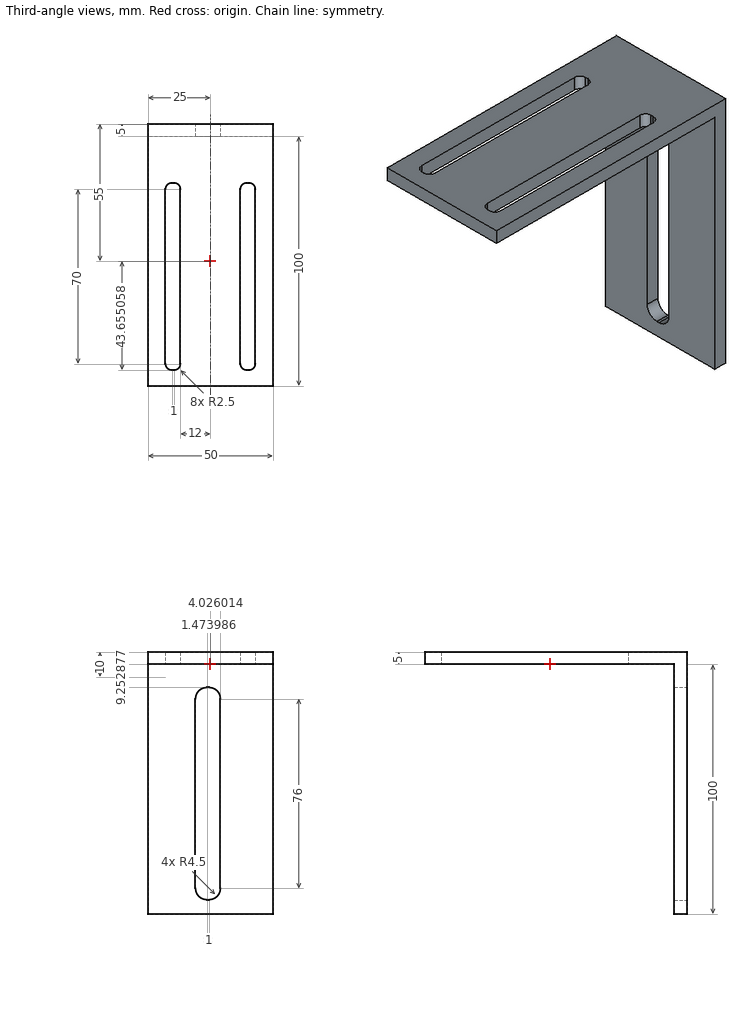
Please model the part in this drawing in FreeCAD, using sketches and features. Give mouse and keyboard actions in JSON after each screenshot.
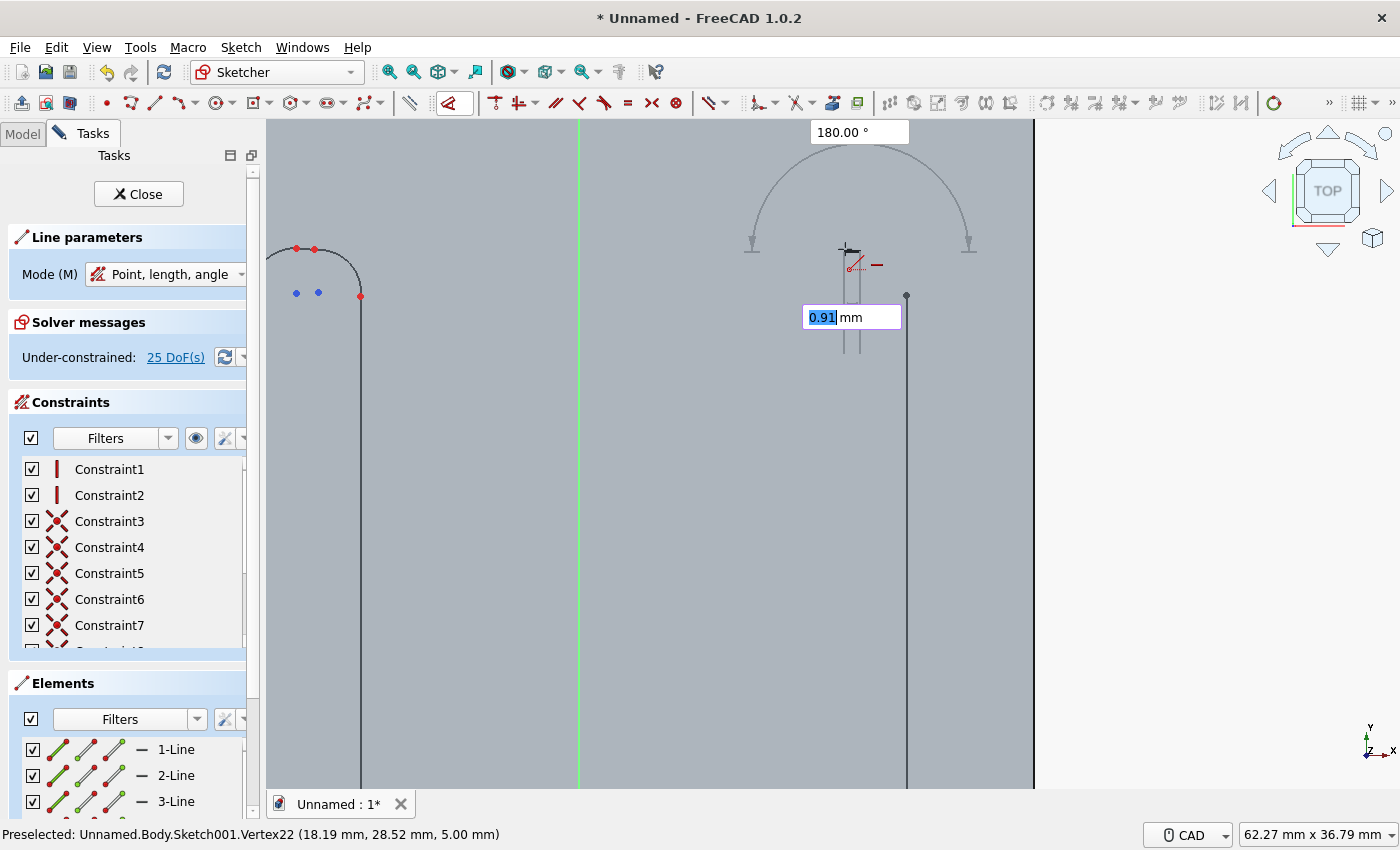
{"action": "left_click", "coordinate": [843, 249]}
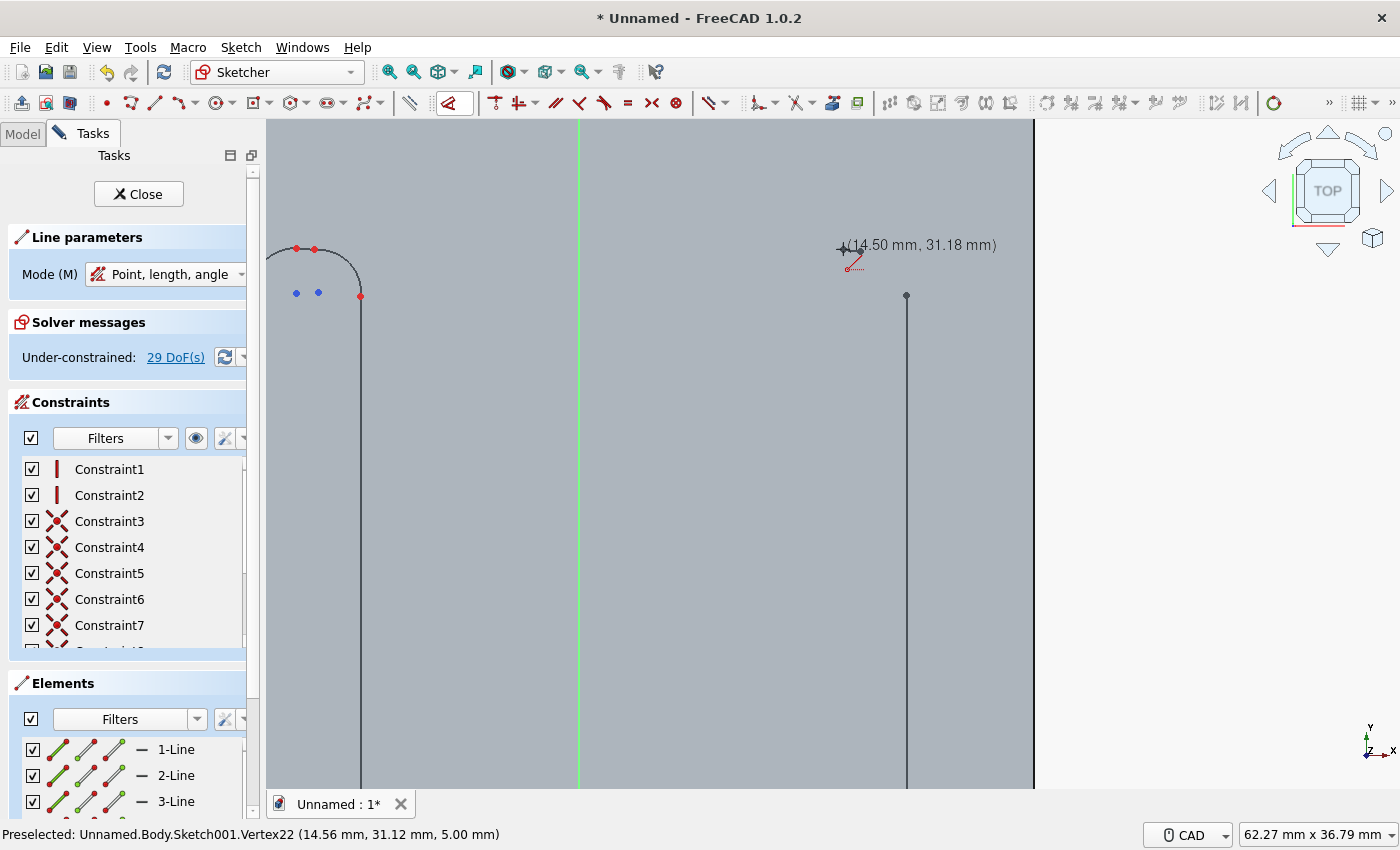
{"action": "left_click", "coordinate": [797, 292]}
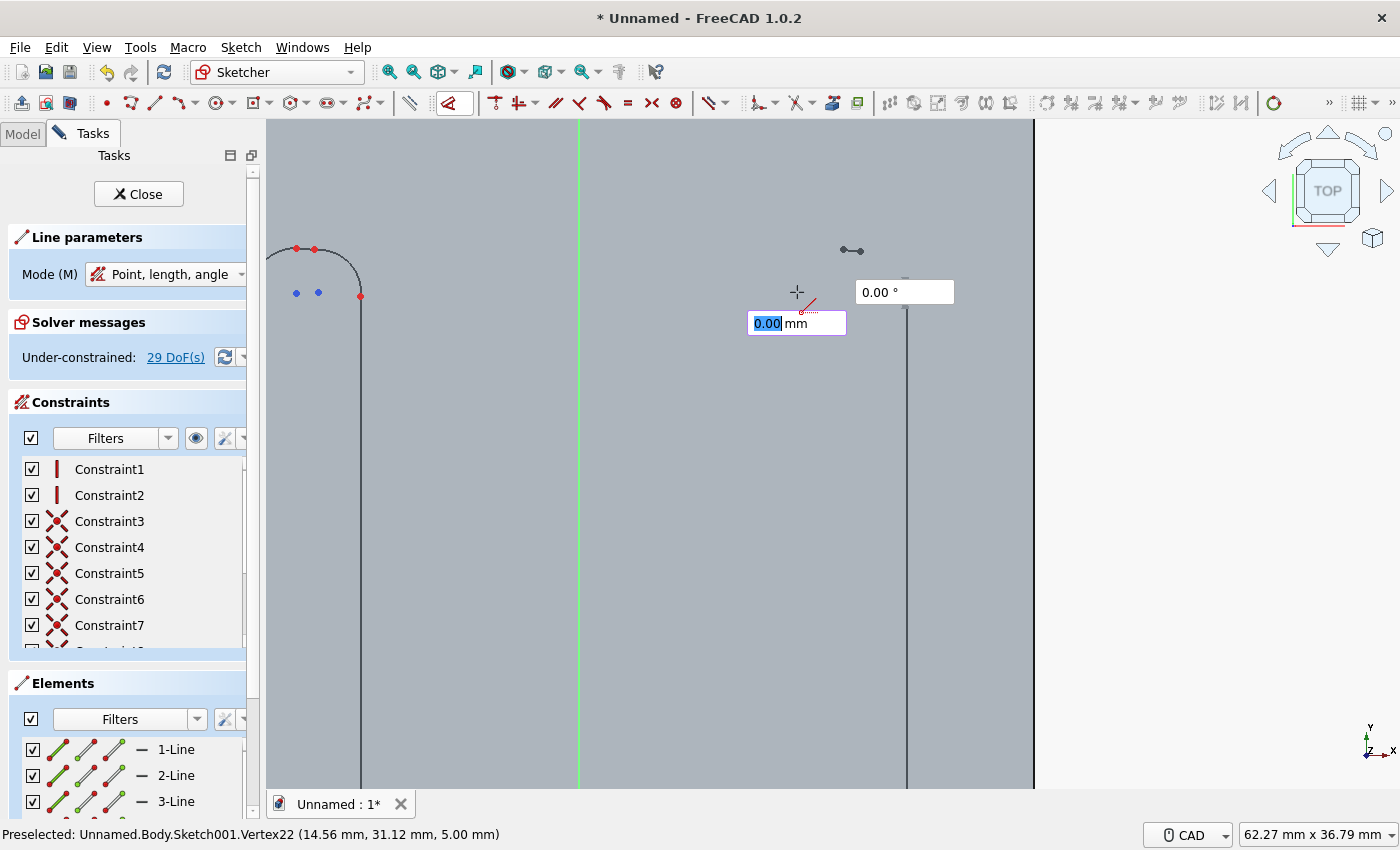
{"action": "scroll", "coordinate": [844, 249], "scroll_direction": "down", "scroll_amount": 6}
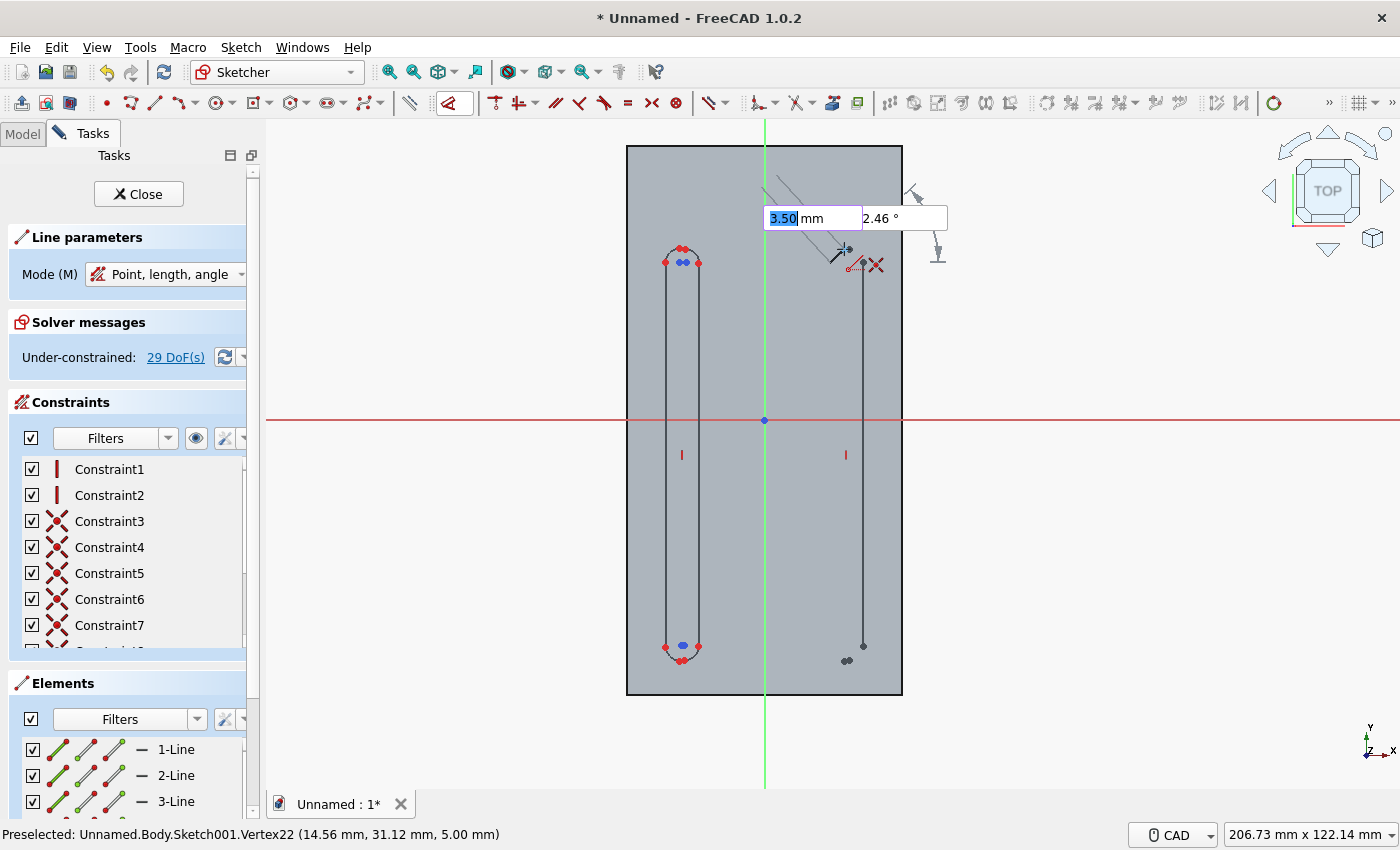
{"action": "left_click", "coordinate": [830, 646]}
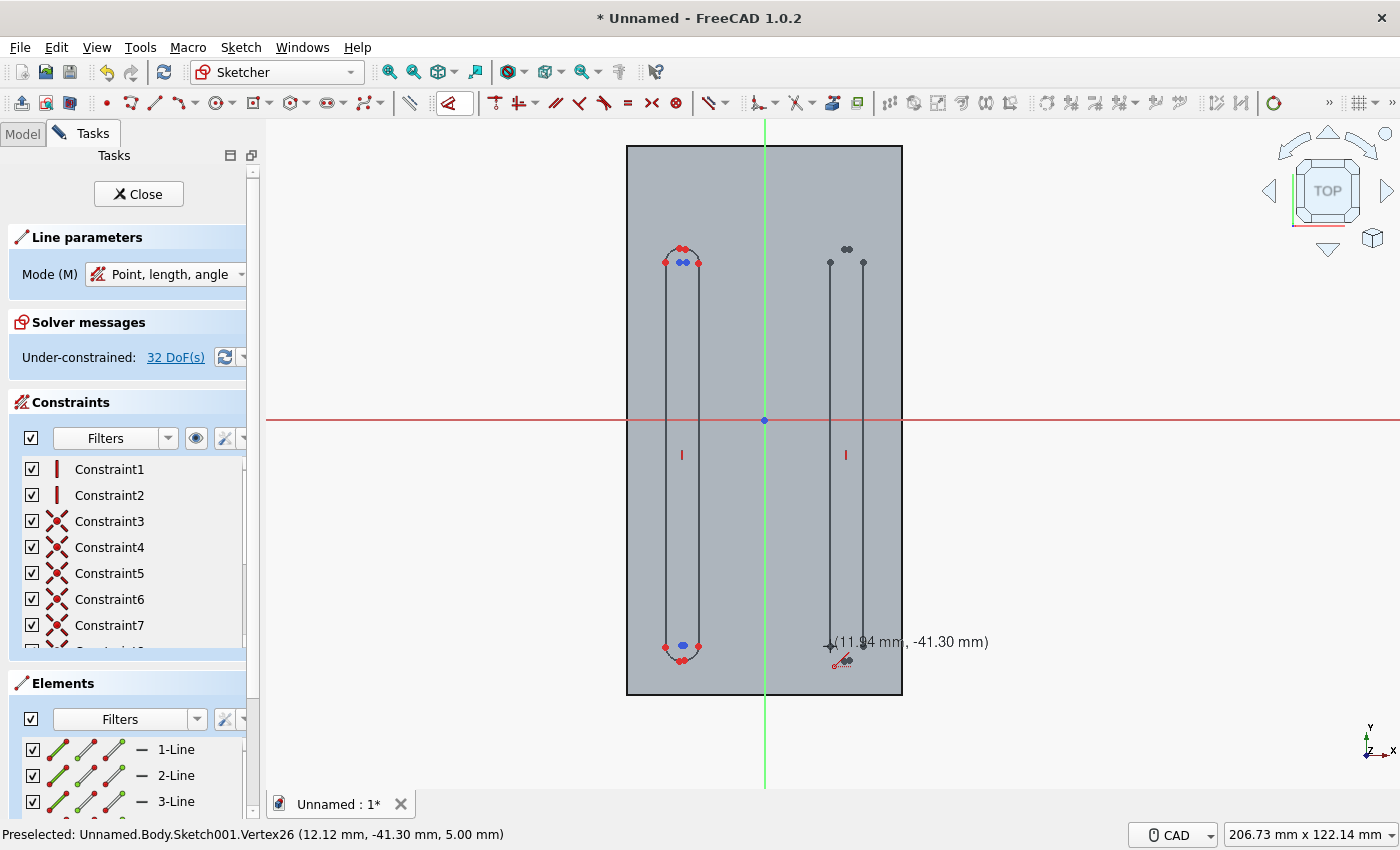
{"action": "key", "text": "g 3 a"}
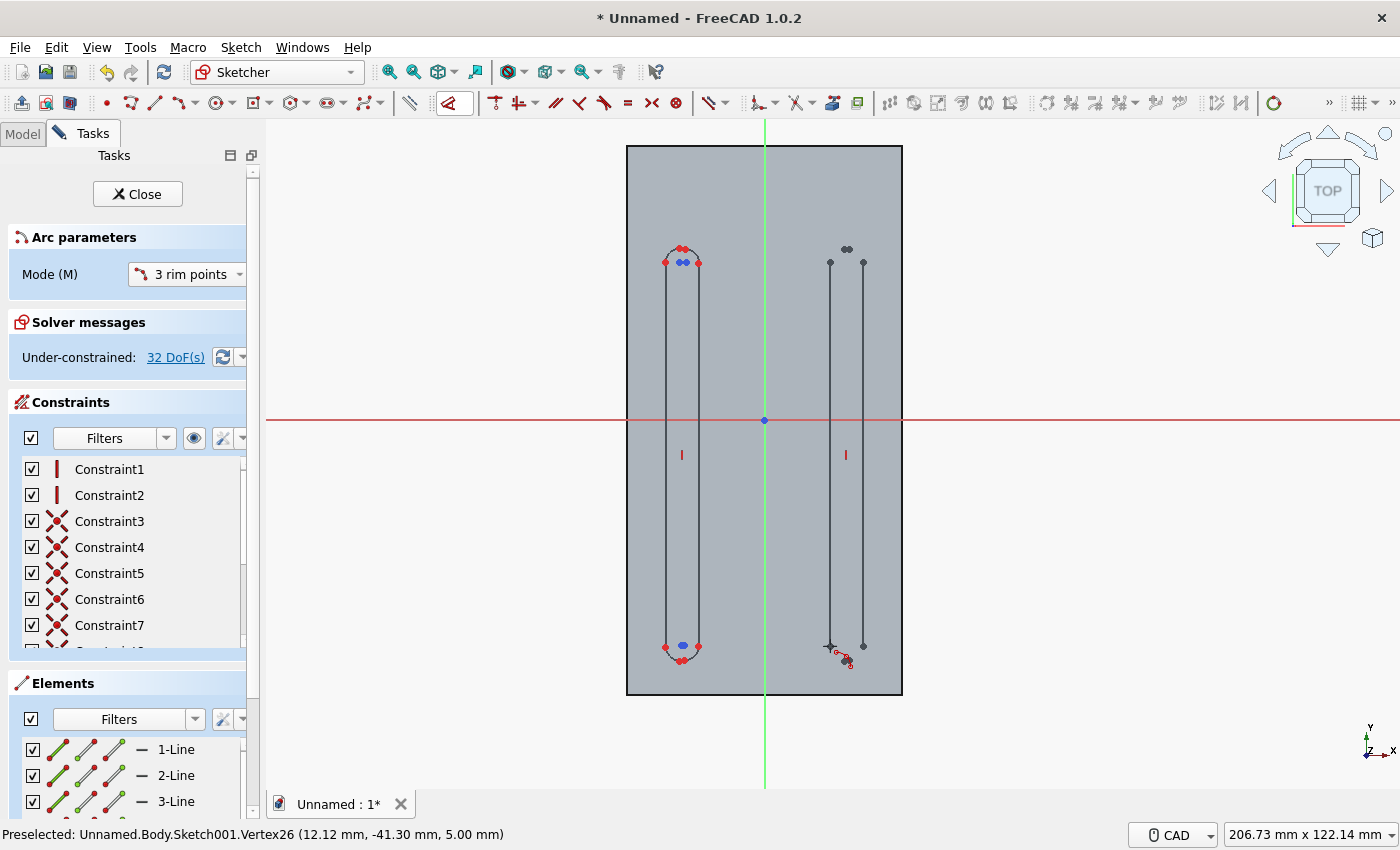
{"action": "scroll", "coordinate": [850, 660], "scroll_direction": "up", "scroll_amount": 9}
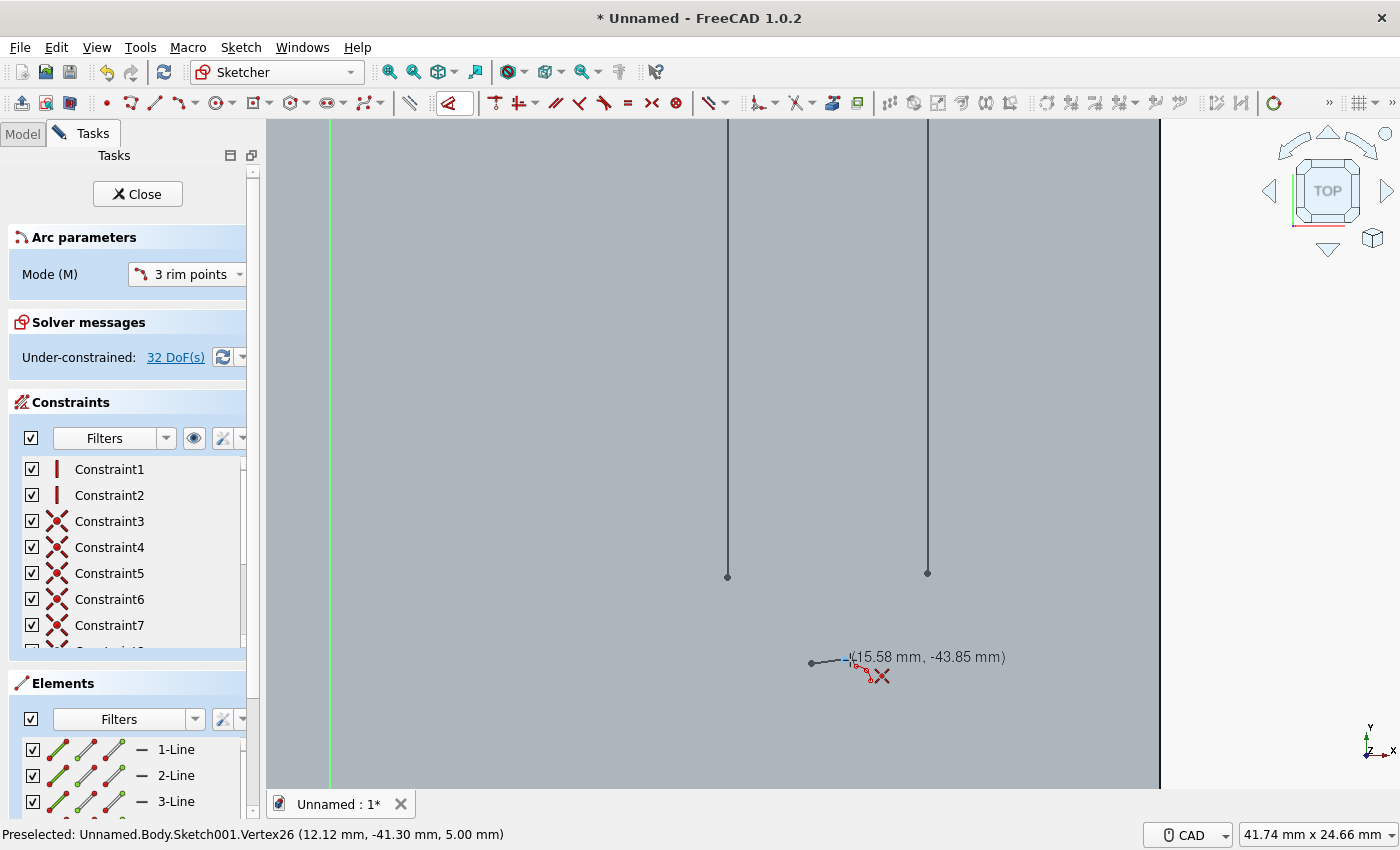
{"action": "left_click", "coordinate": [844, 659]}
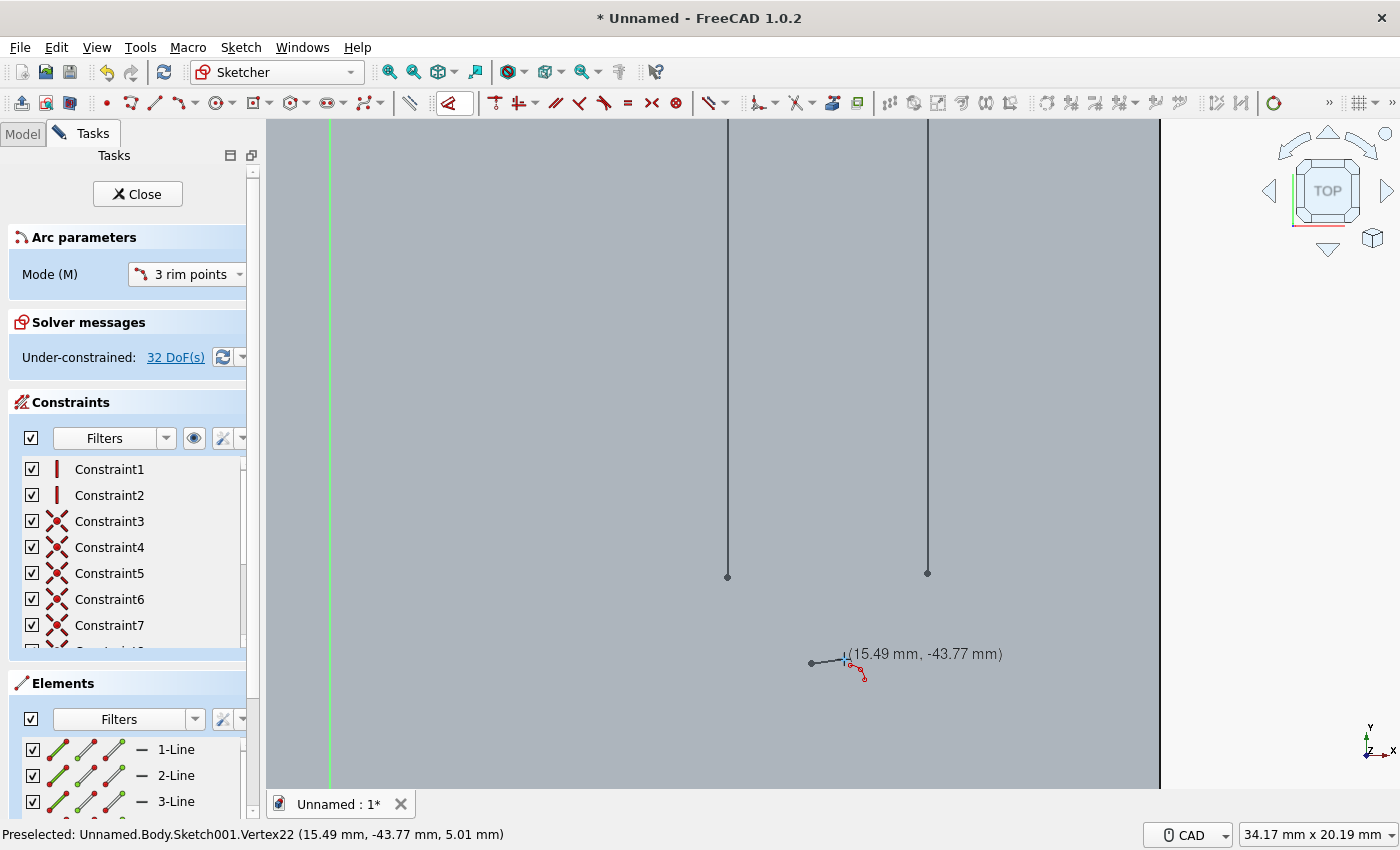
{"action": "scroll", "coordinate": [851, 661], "scroll_direction": "down", "scroll_amount": 9}